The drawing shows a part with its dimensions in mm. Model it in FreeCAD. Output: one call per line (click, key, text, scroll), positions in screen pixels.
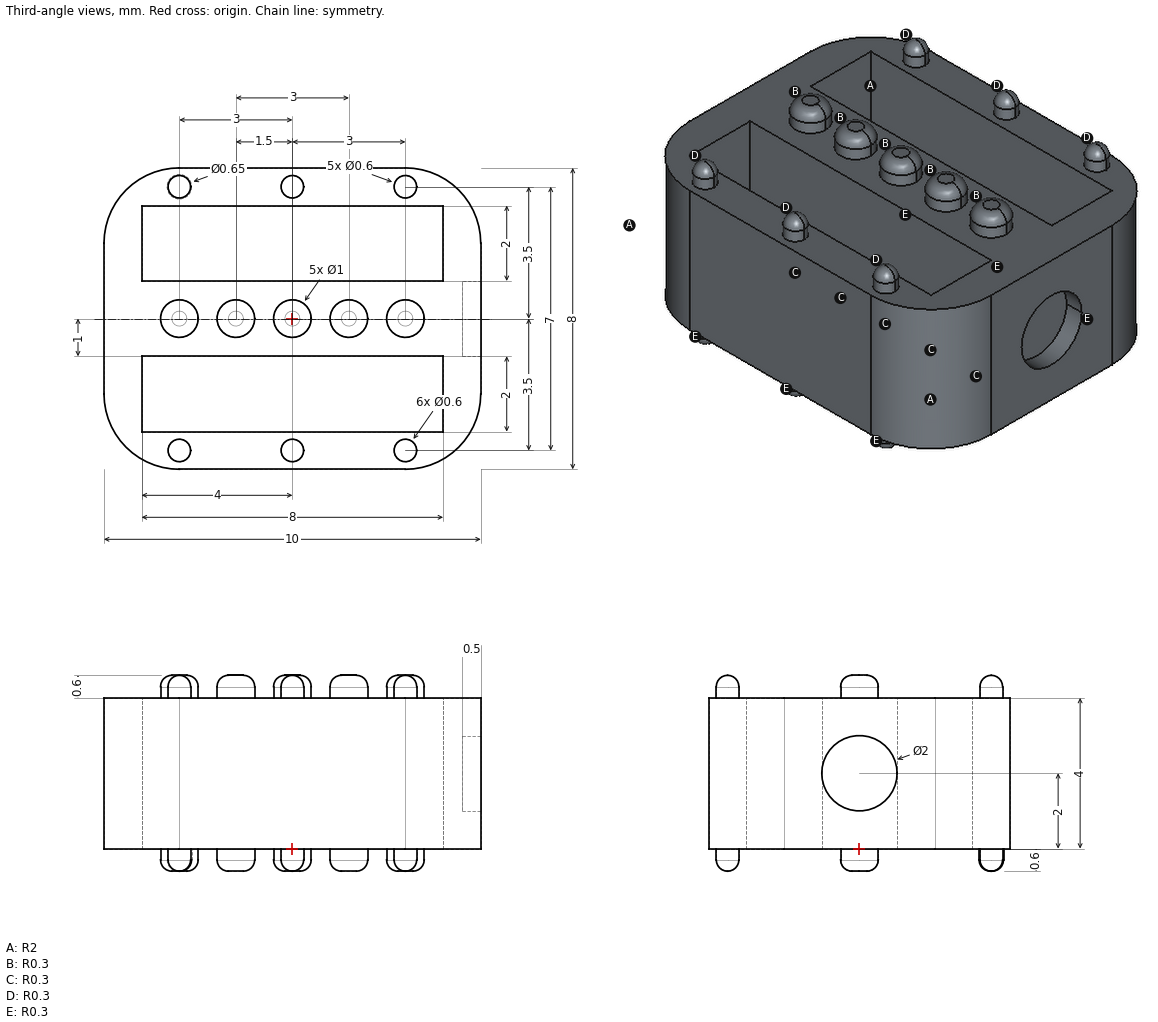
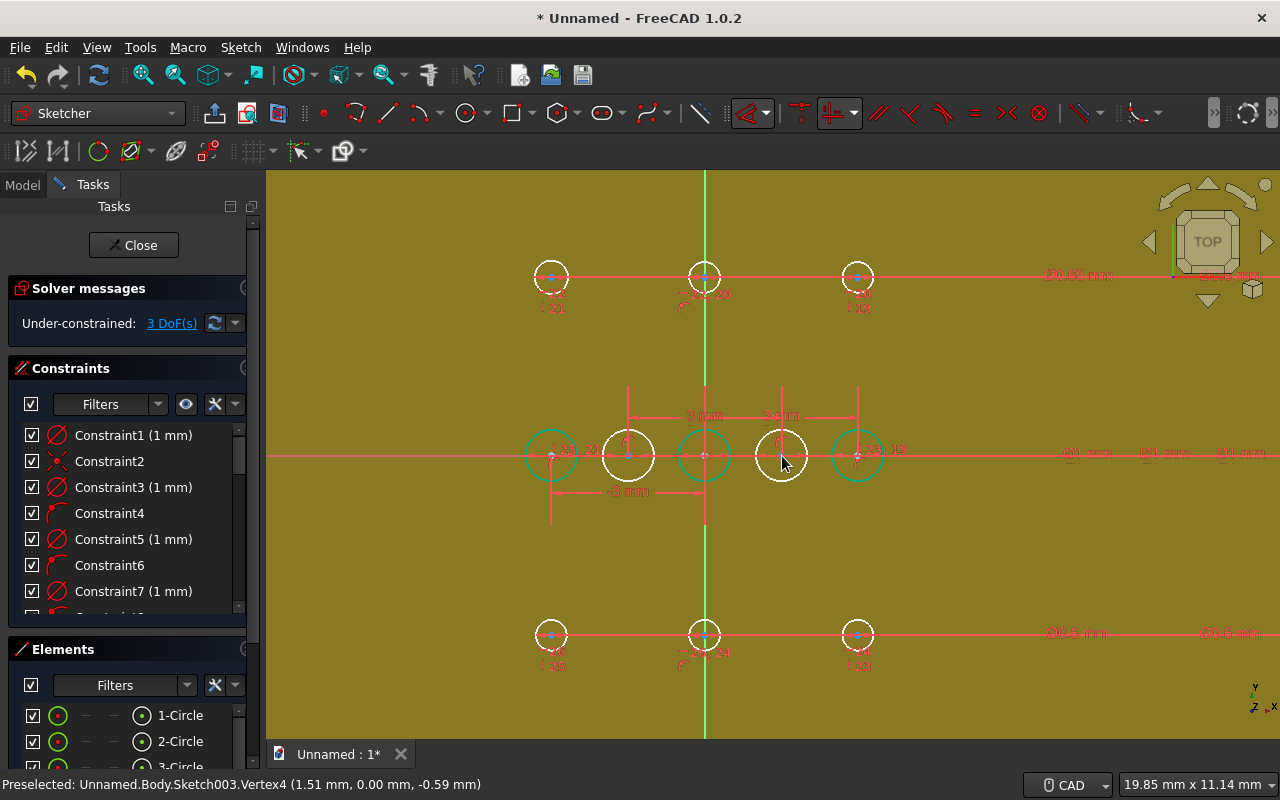
click(858, 277)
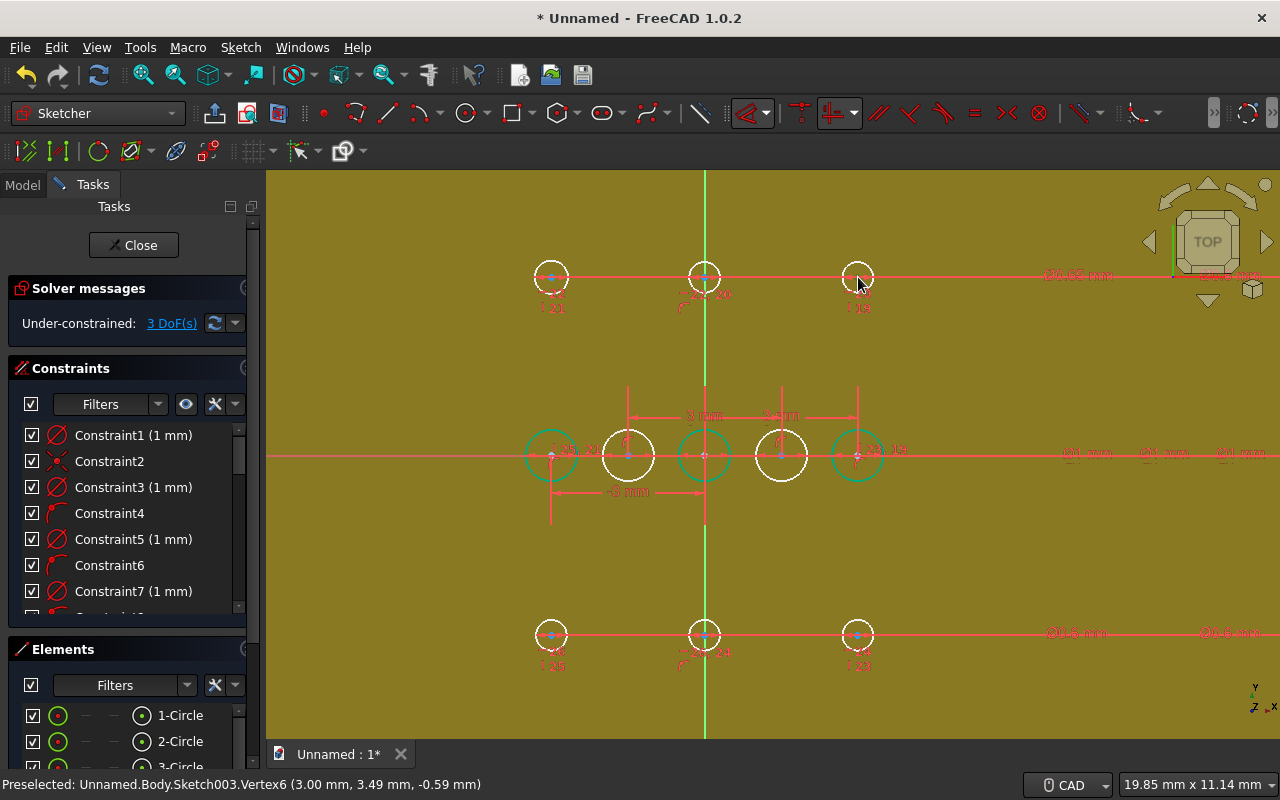
click(858, 635)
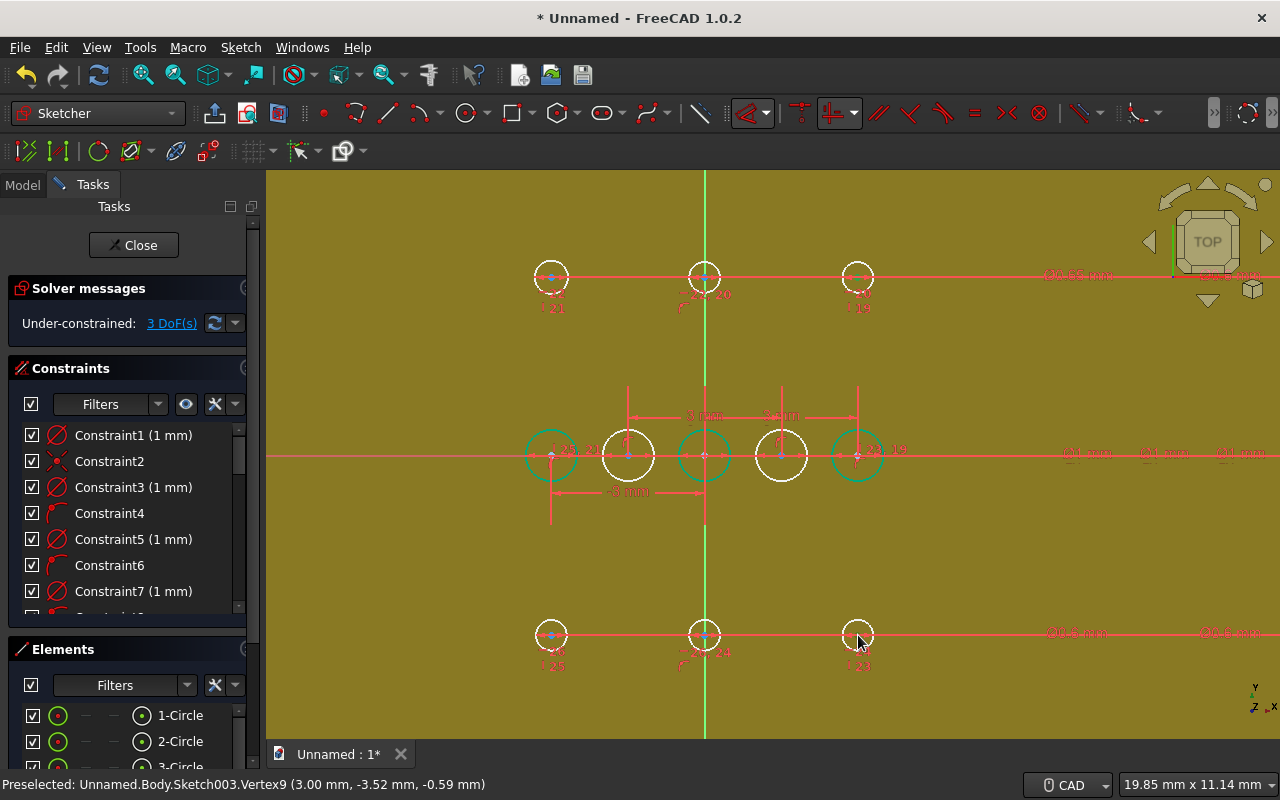
key(i)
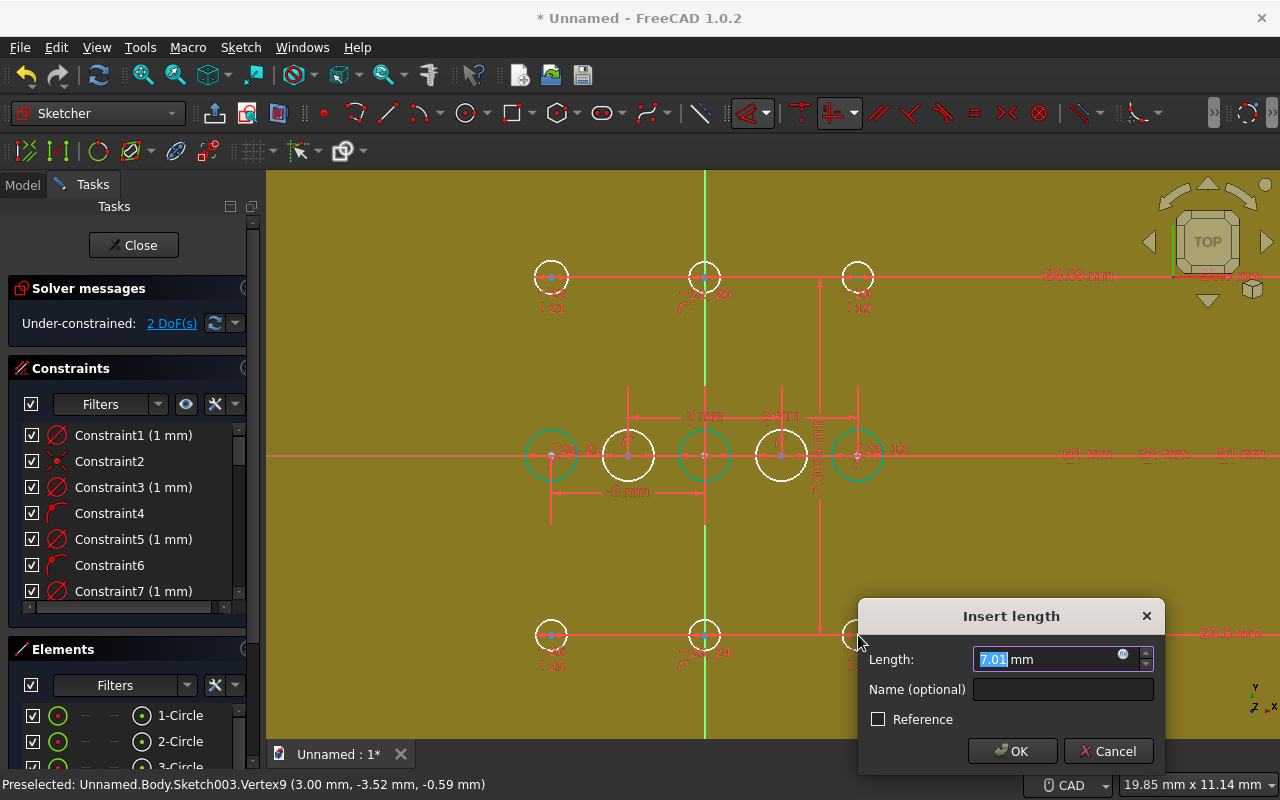
text(7)
key(Return)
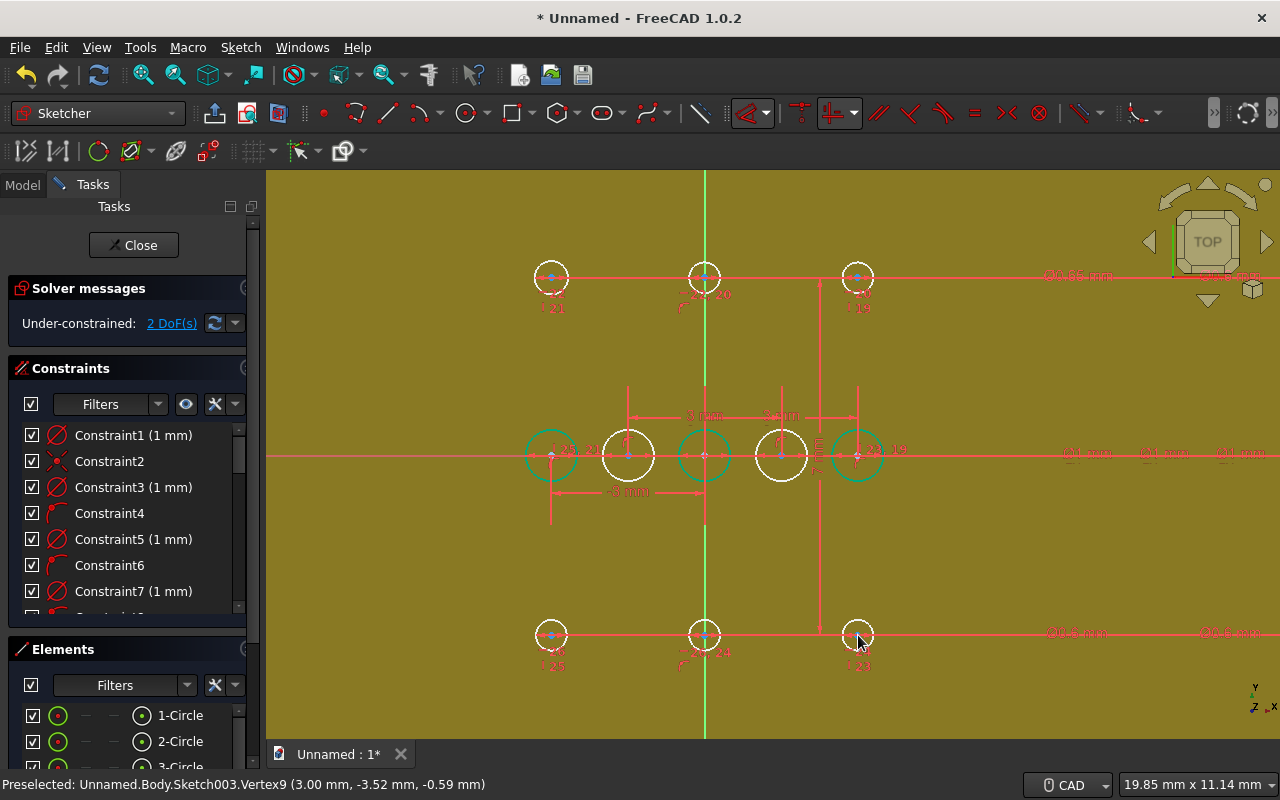
click(628, 456)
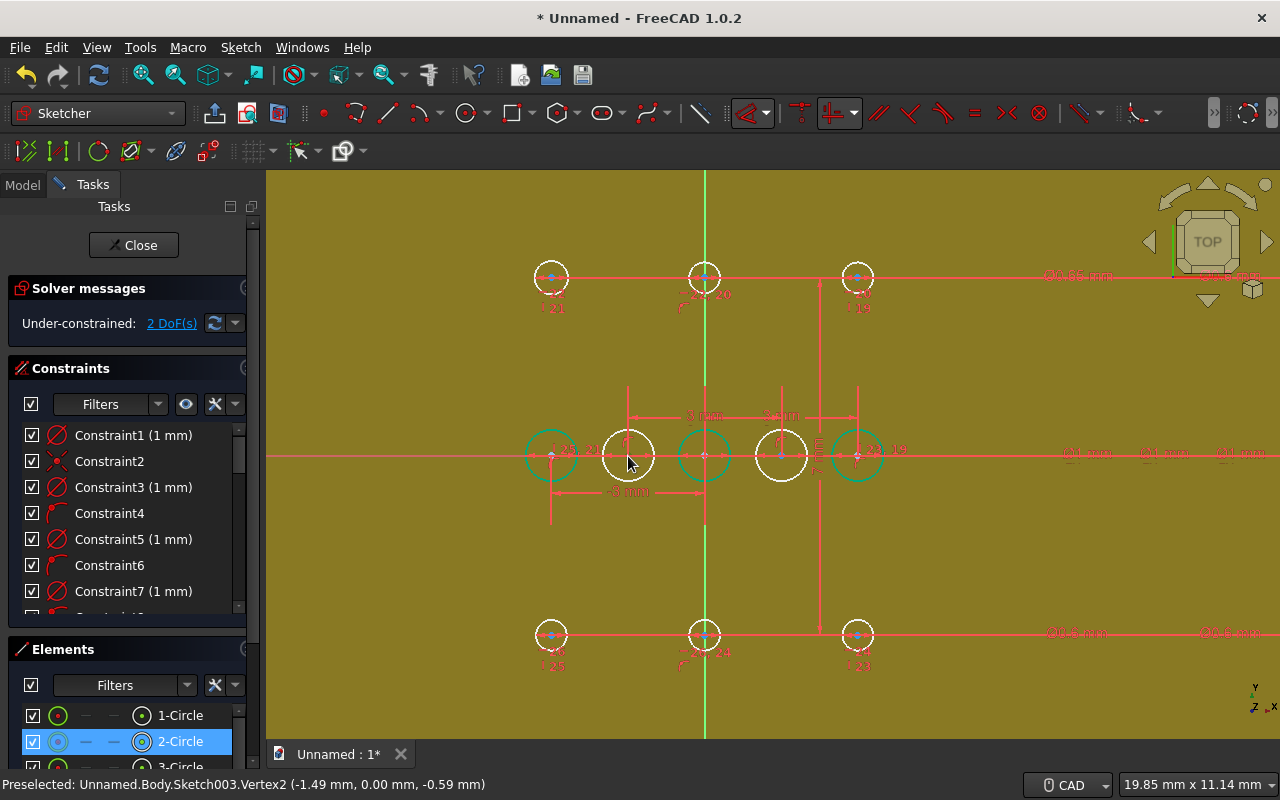
click(768, 114)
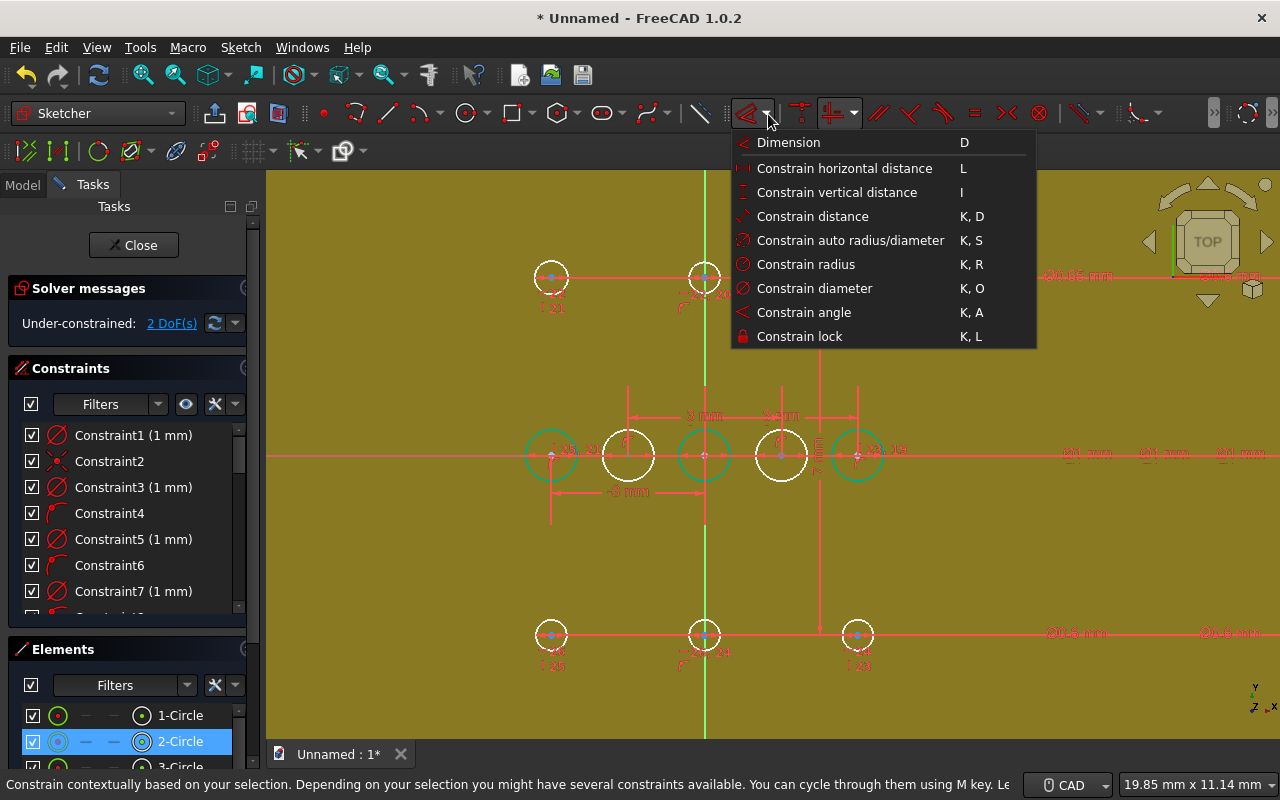
click(884, 168)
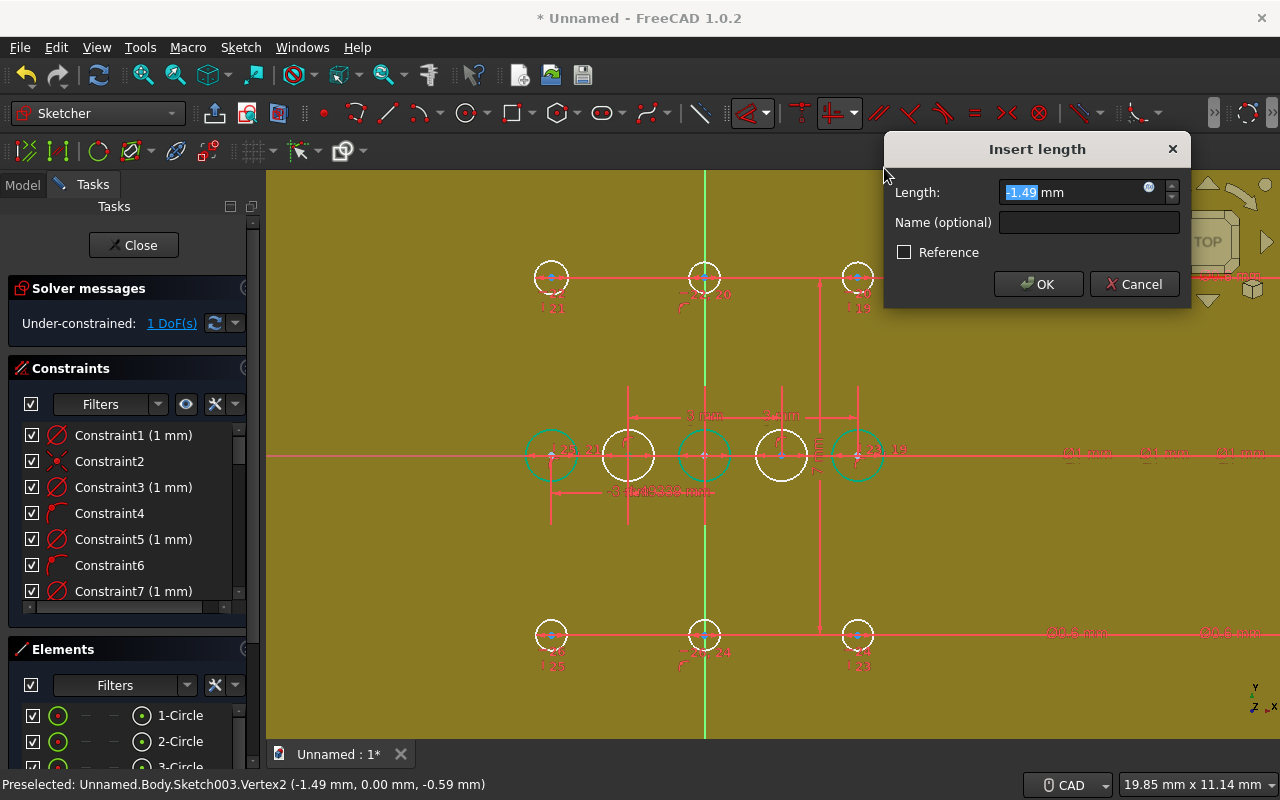
text(-1.5)
key(Return)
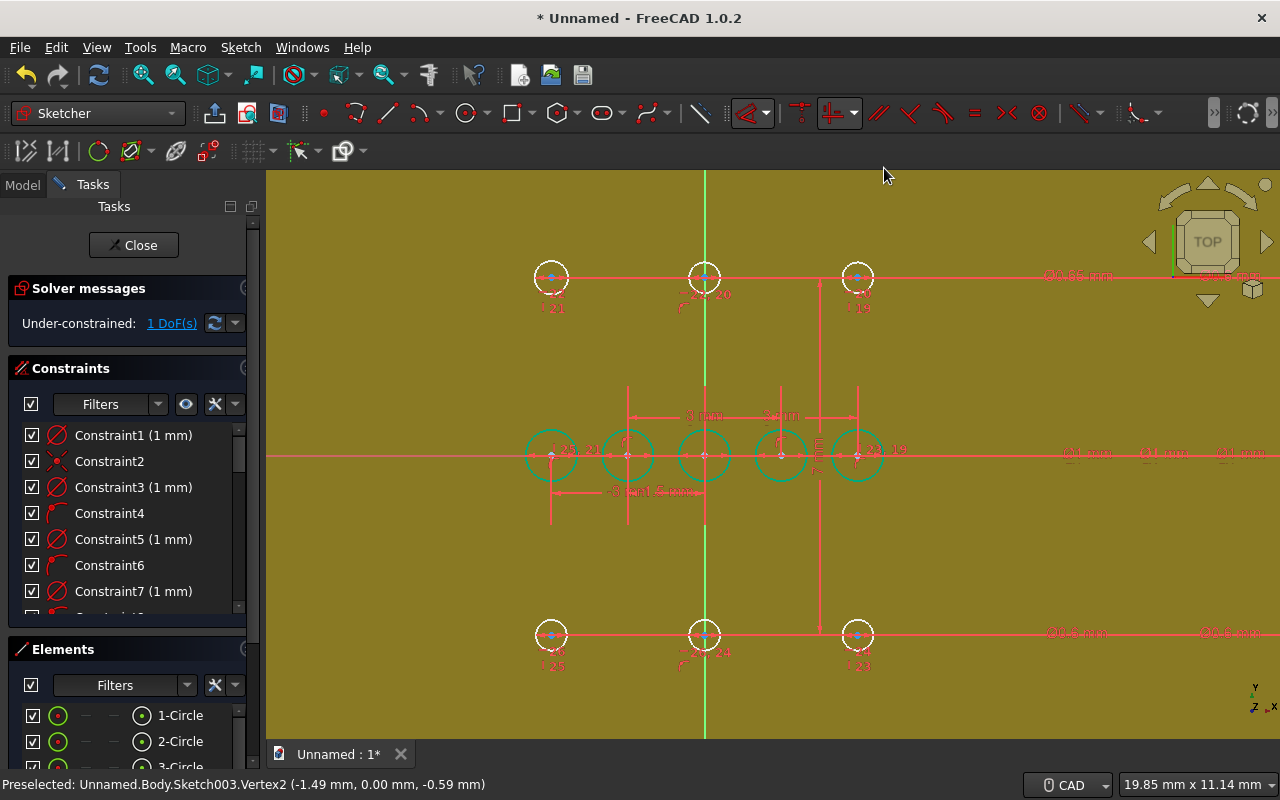
click(858, 278)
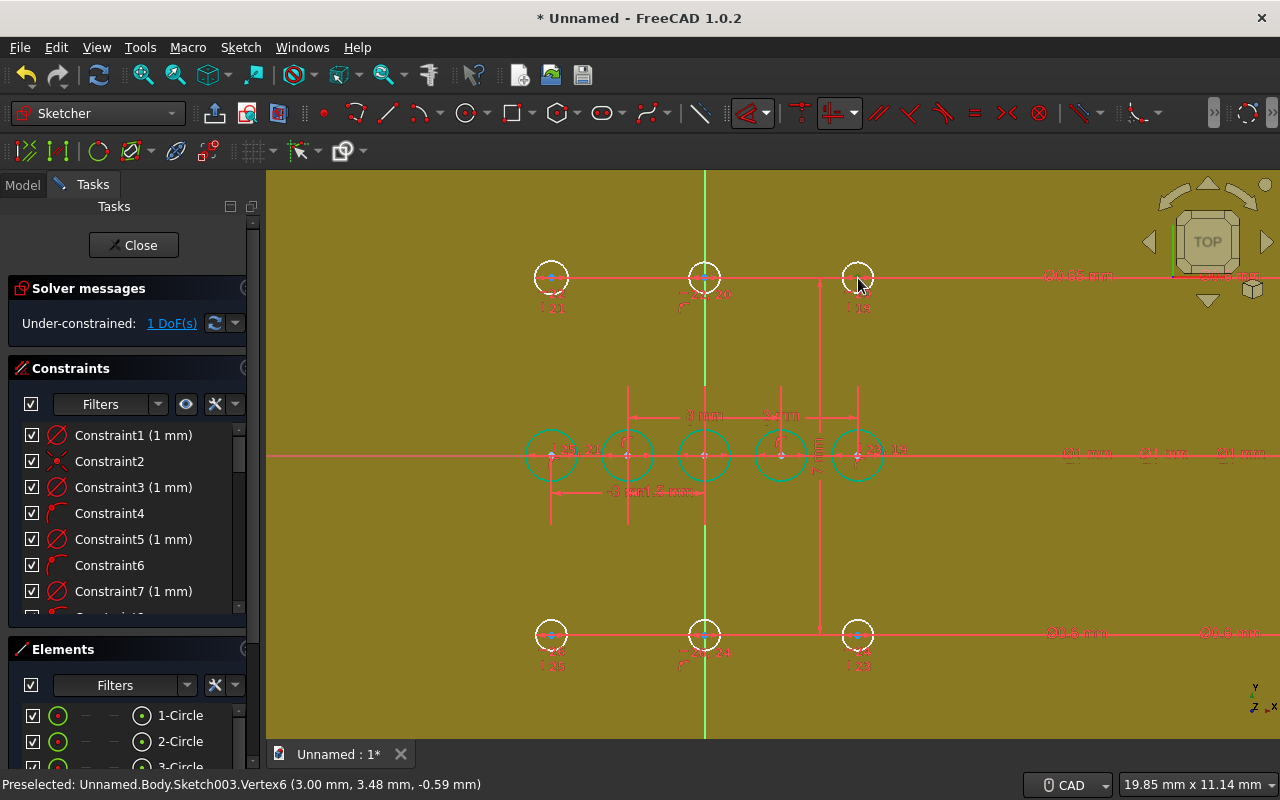
click(768, 114)